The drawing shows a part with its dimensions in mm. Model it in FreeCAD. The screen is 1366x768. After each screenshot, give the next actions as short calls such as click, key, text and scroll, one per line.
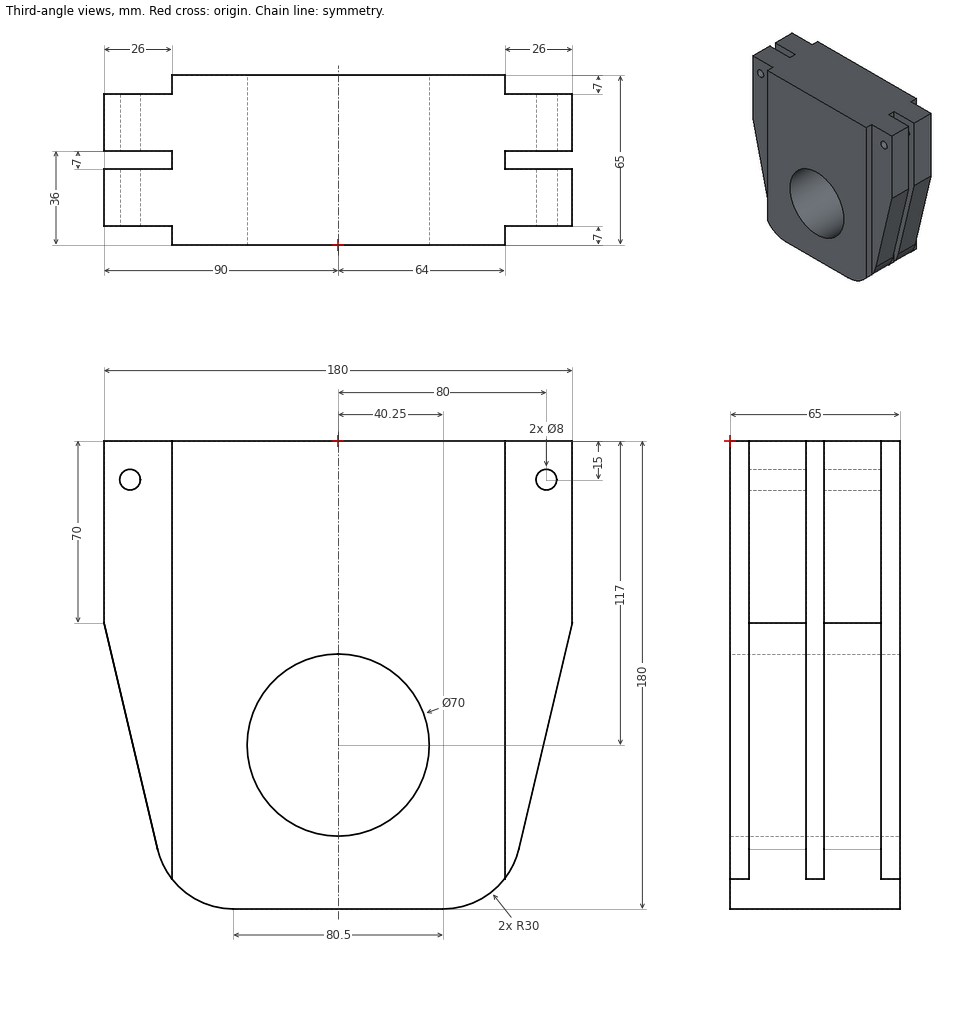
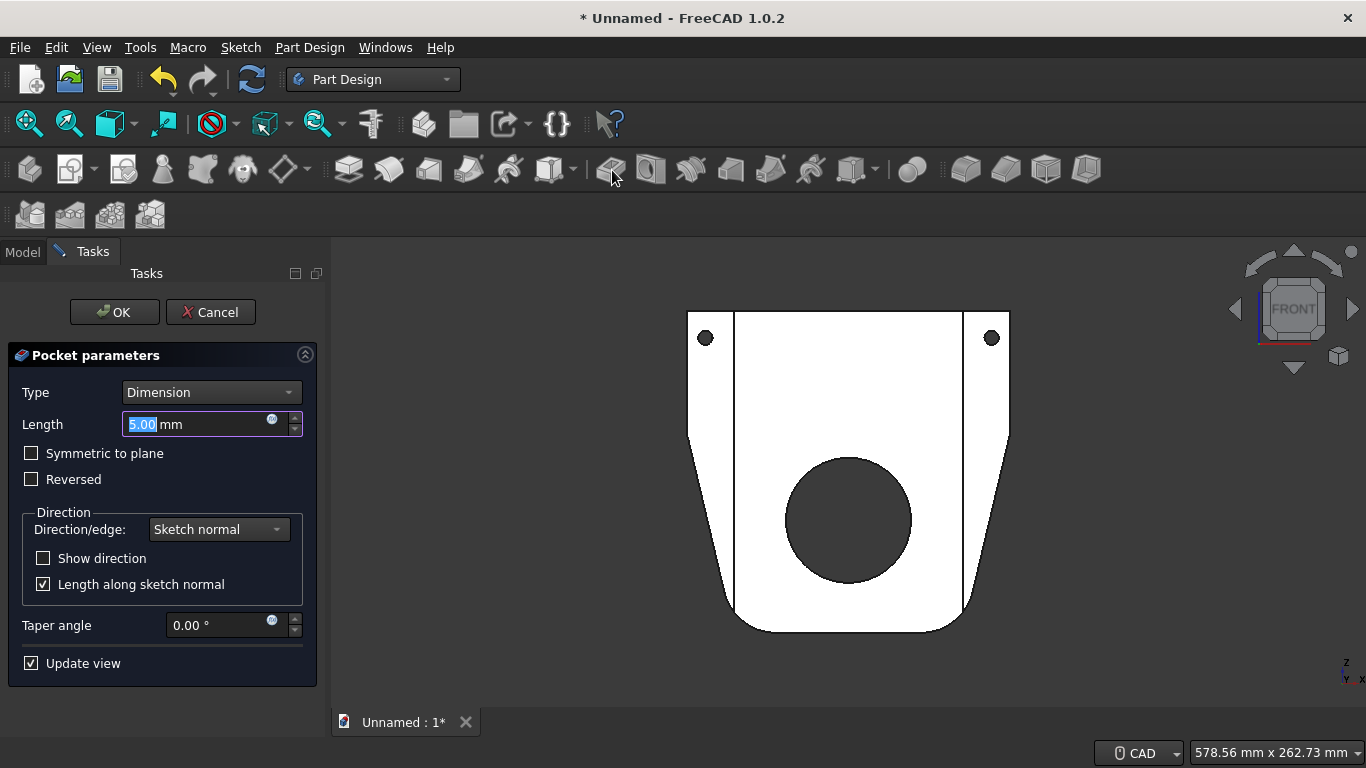
click(212, 392)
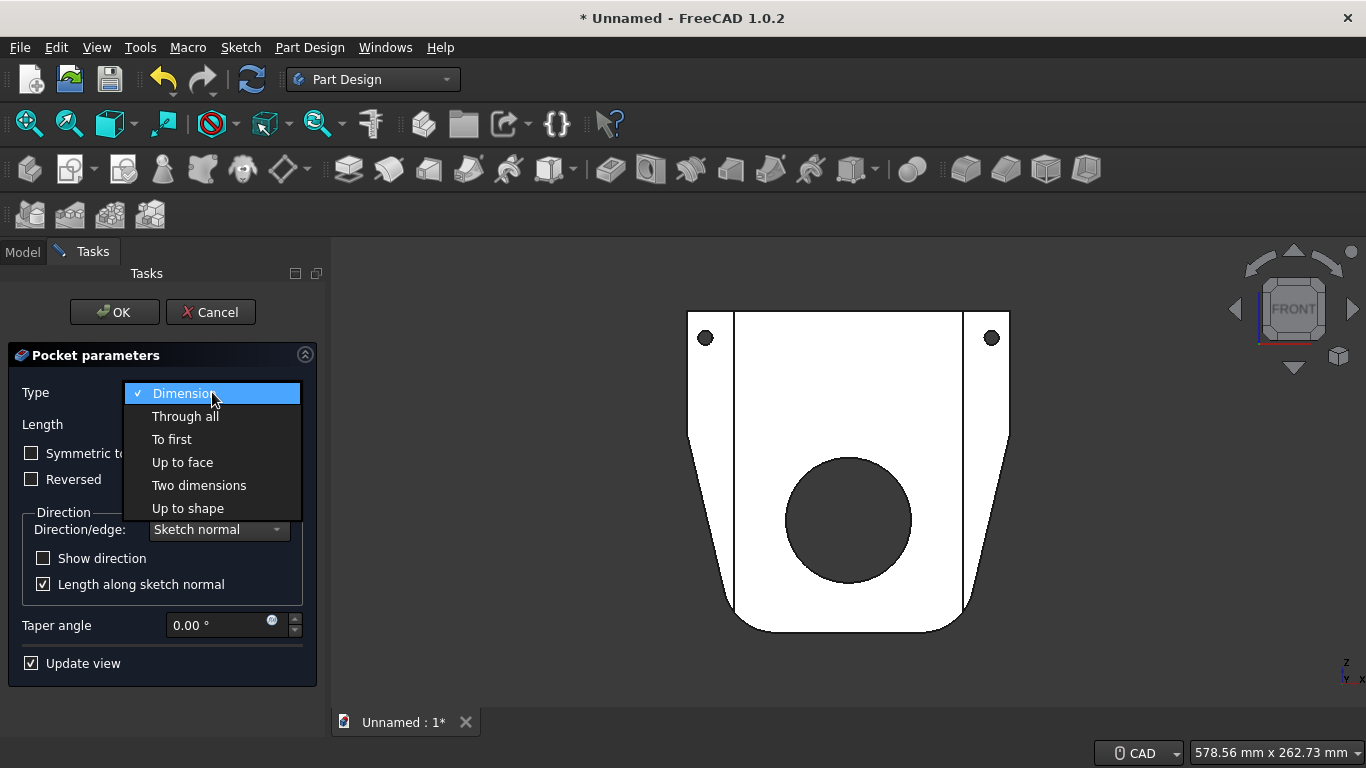
click(212, 416)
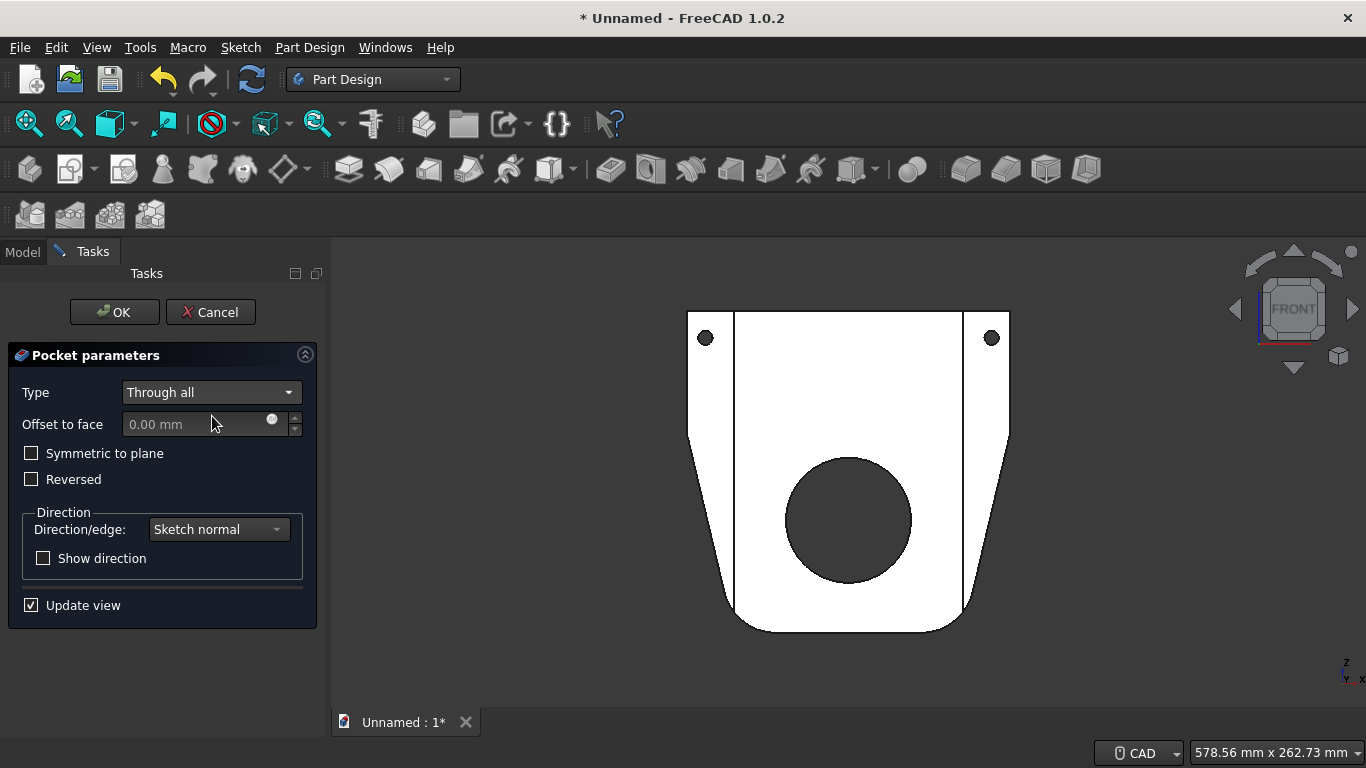
click(115, 312)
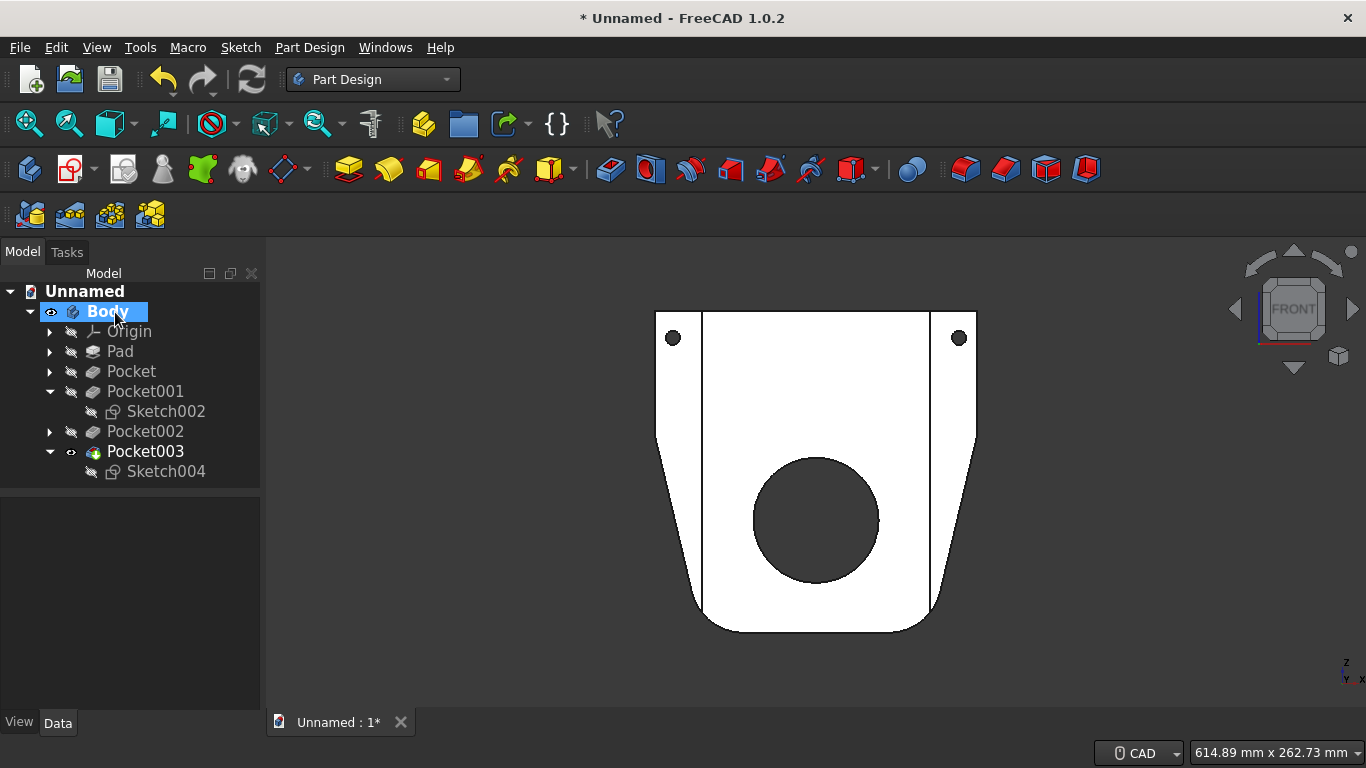
key(0)